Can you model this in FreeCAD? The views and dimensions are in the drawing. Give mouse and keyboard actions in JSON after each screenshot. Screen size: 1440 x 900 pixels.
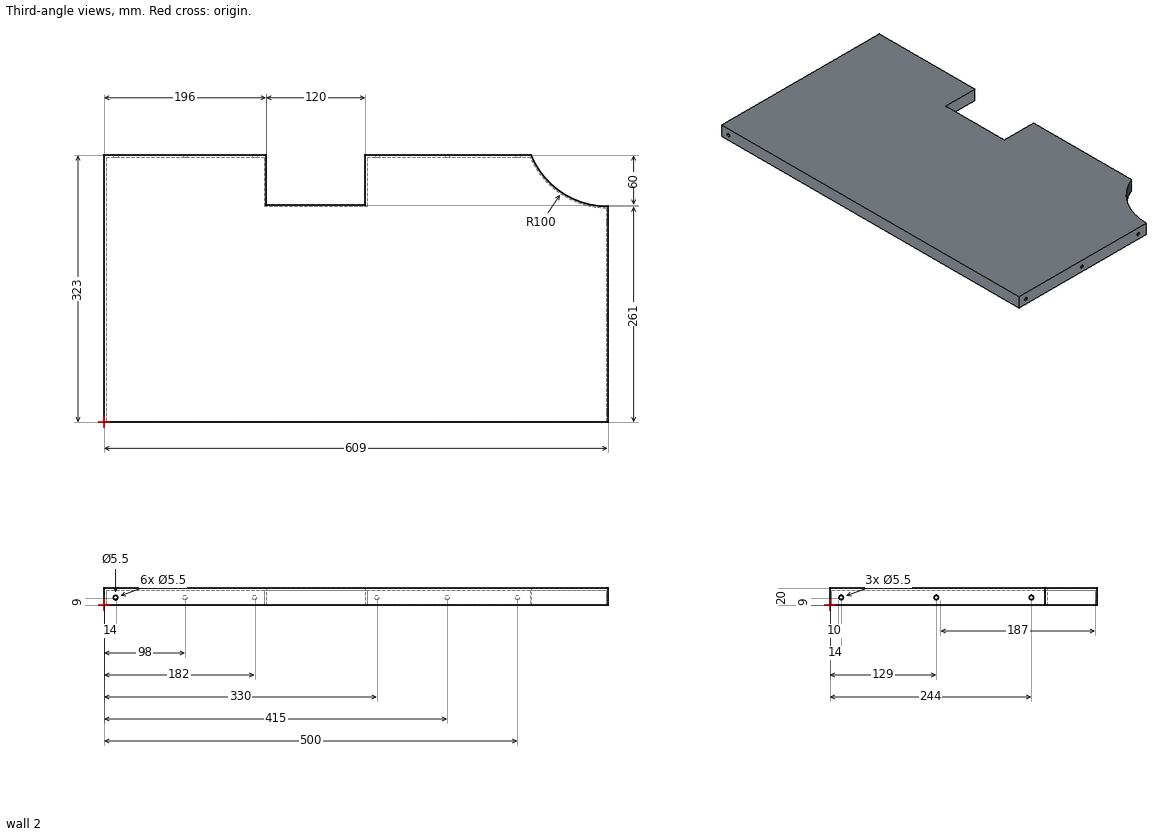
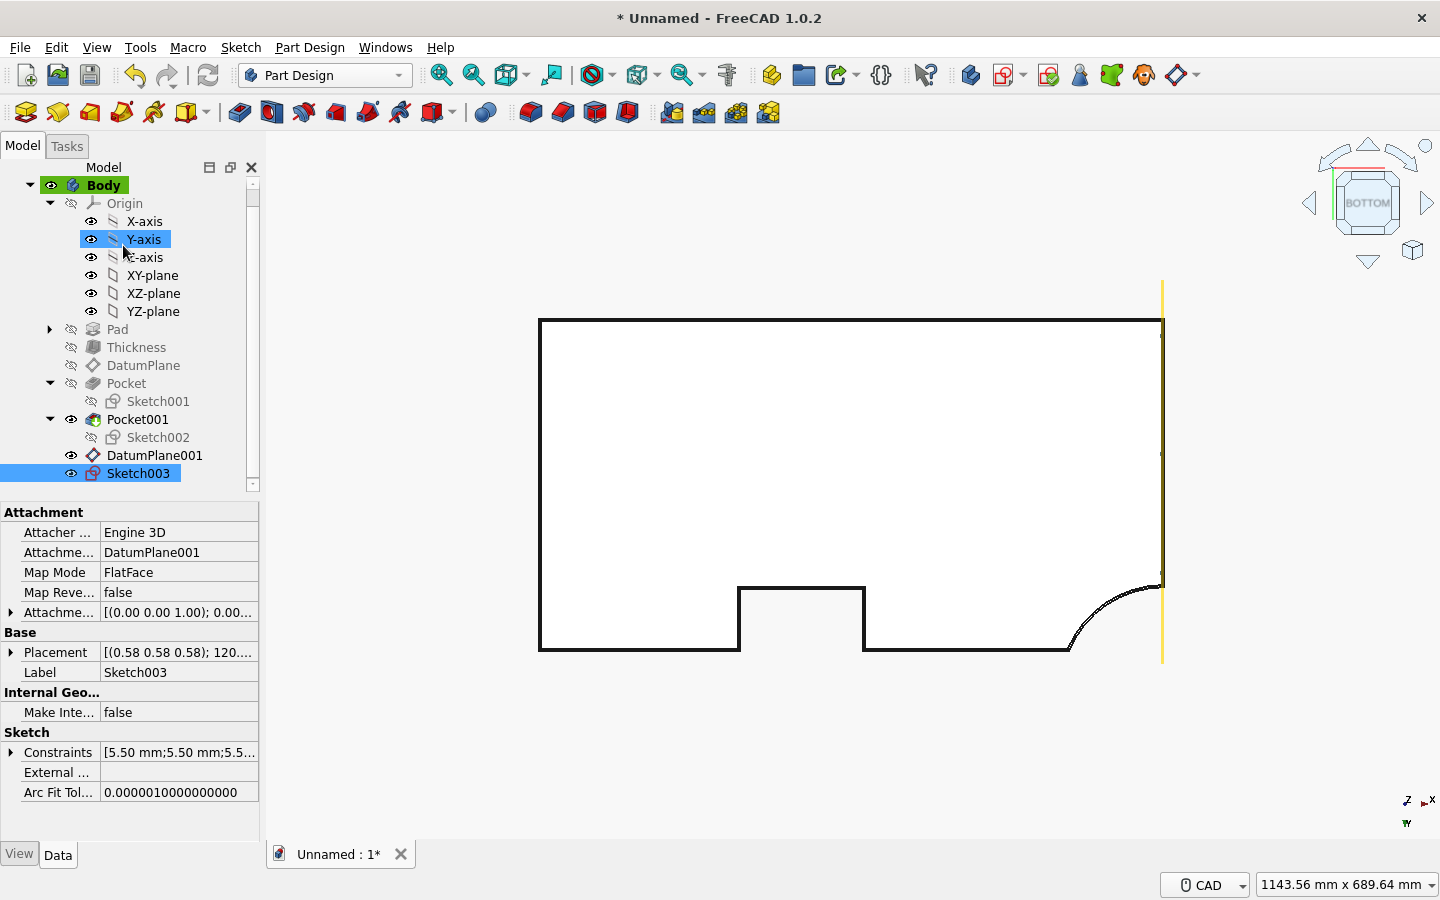
{"action": "left_click", "coordinate": [240, 112]}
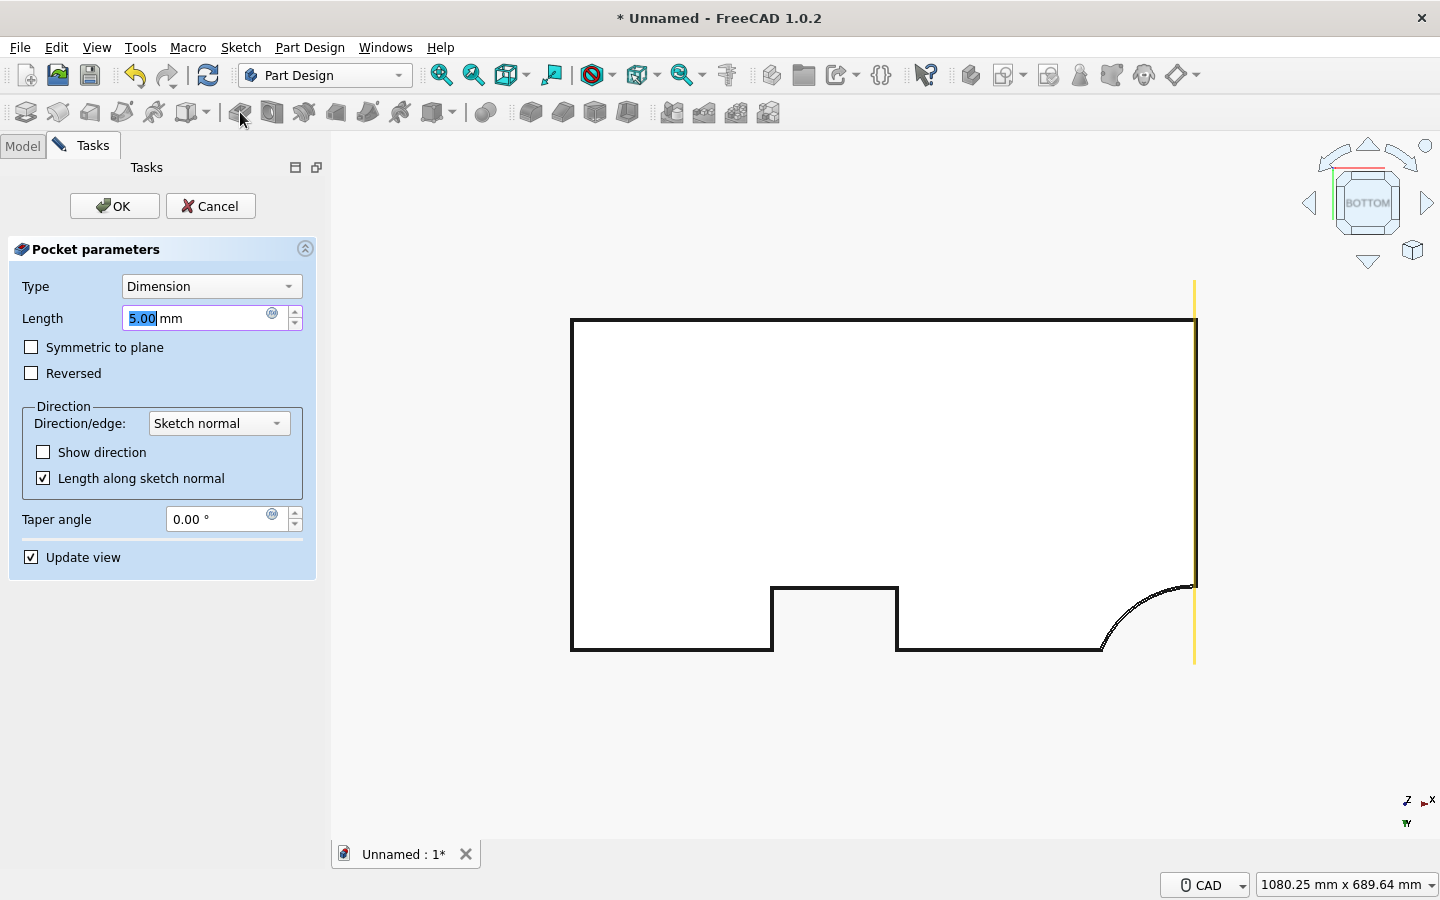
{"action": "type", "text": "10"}
{"action": "key", "text": "Tab"}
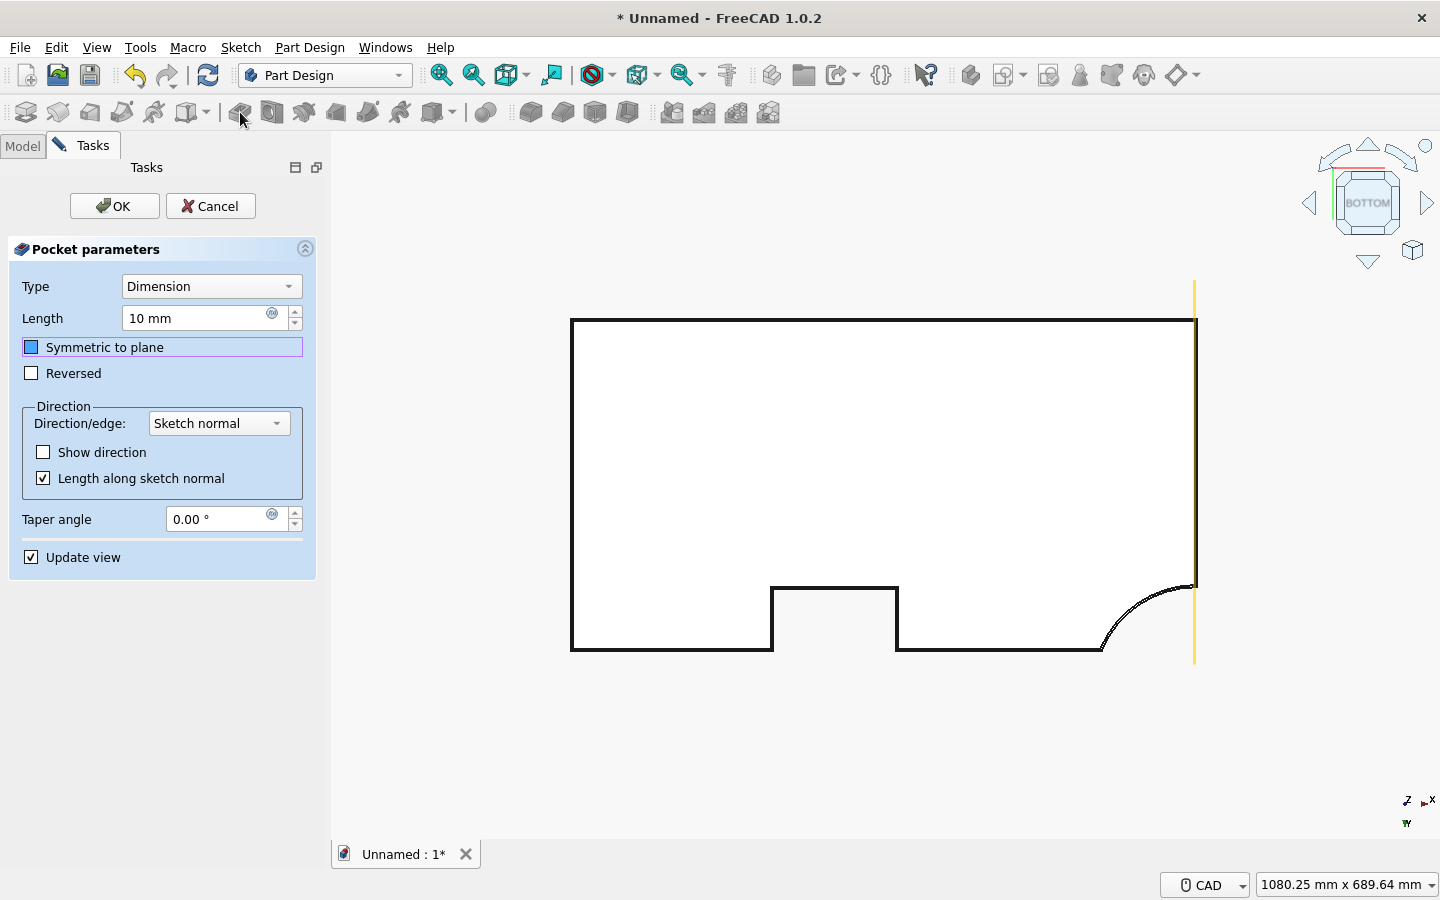
{"action": "left_click", "coordinate": [30, 373]}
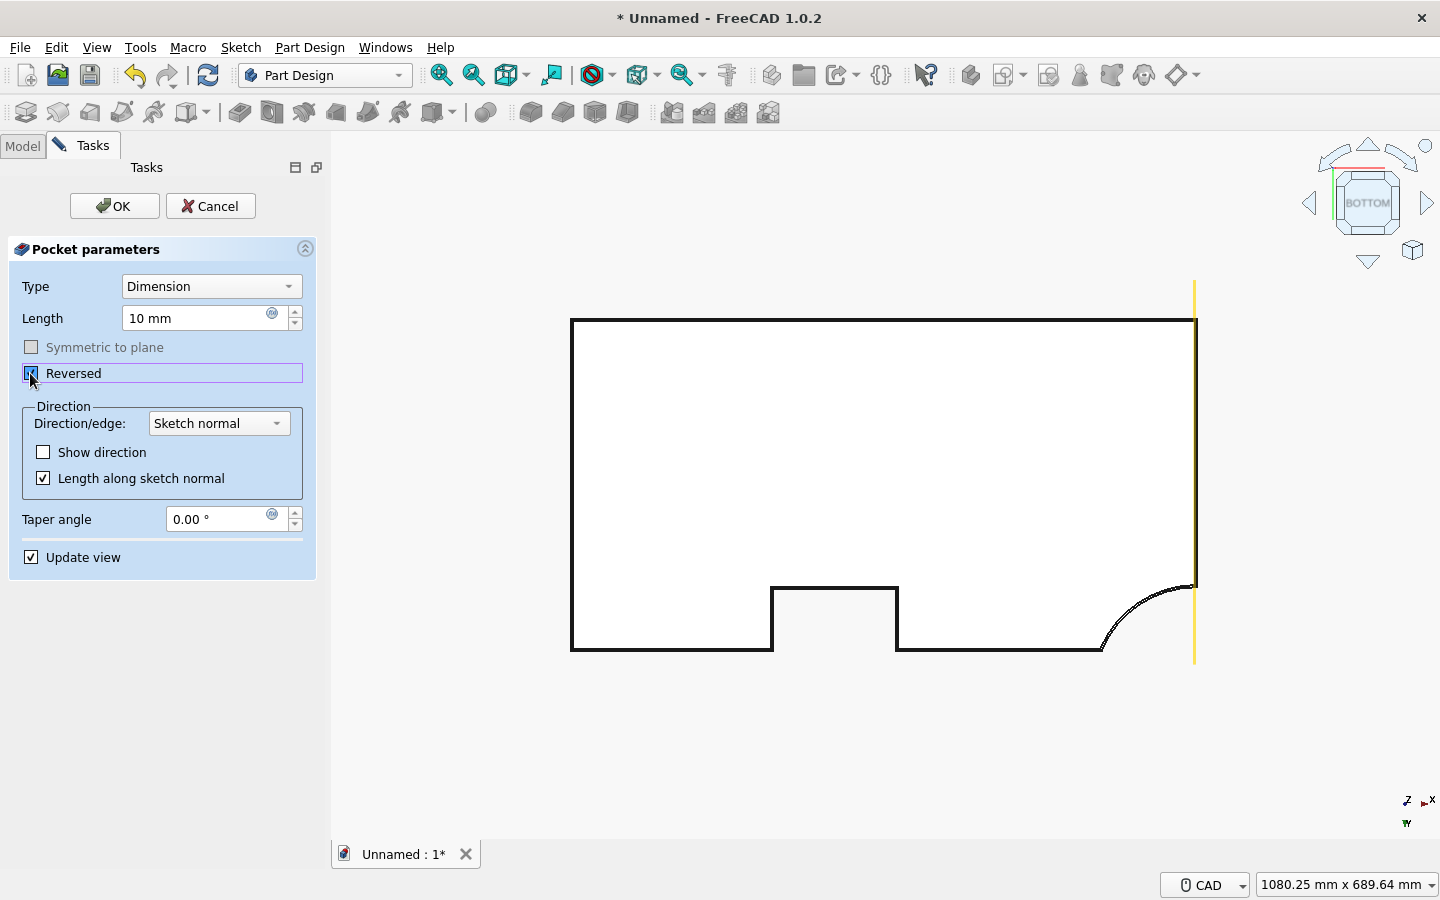
{"action": "left_click", "coordinate": [115, 206]}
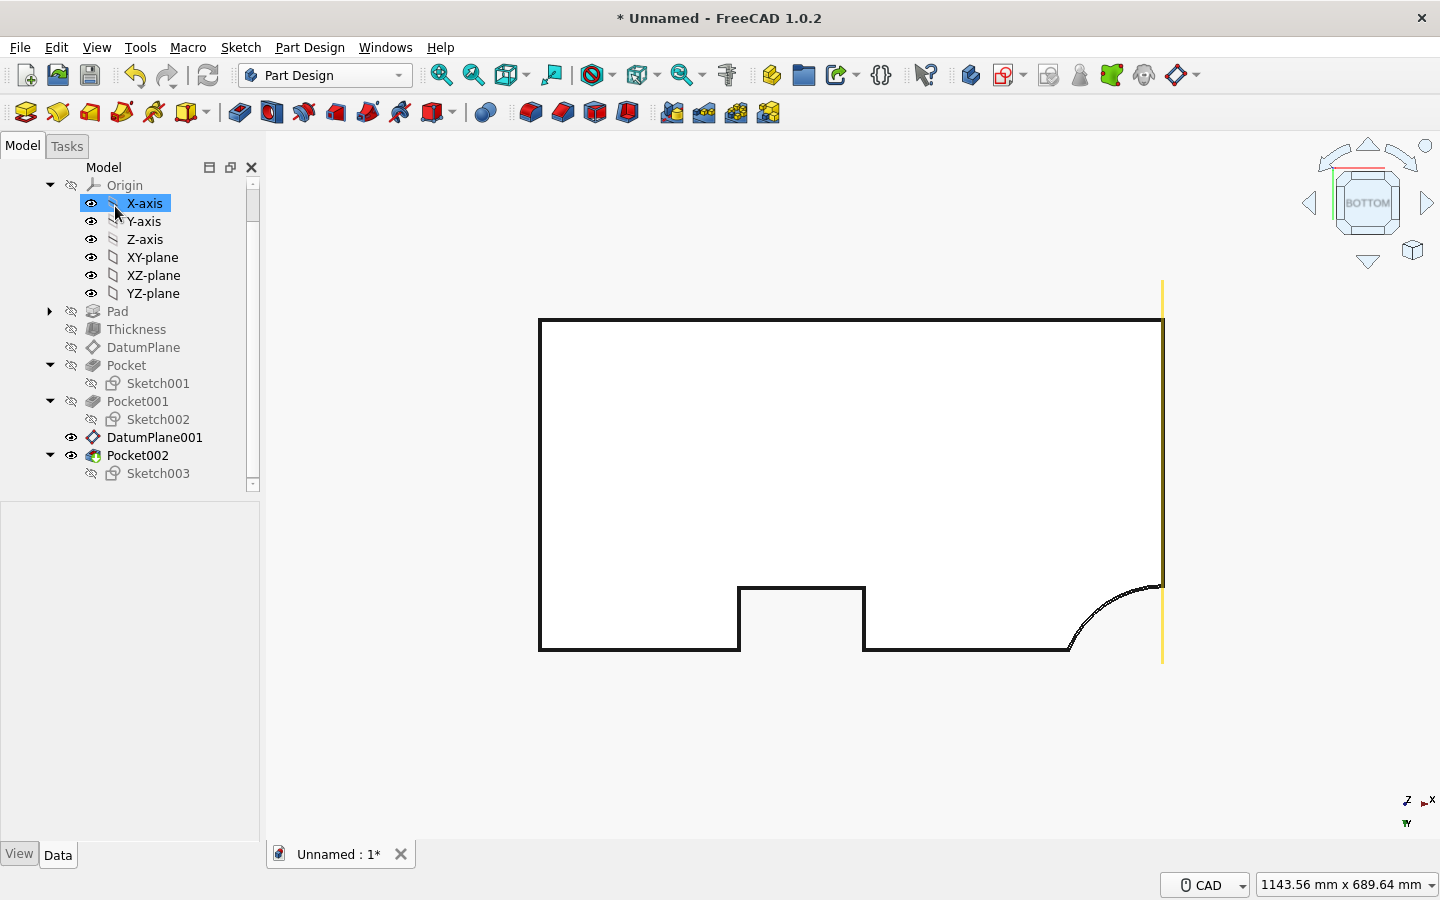
{"action": "left_click", "coordinate": [116, 437]}
{"action": "key", "text": "space"}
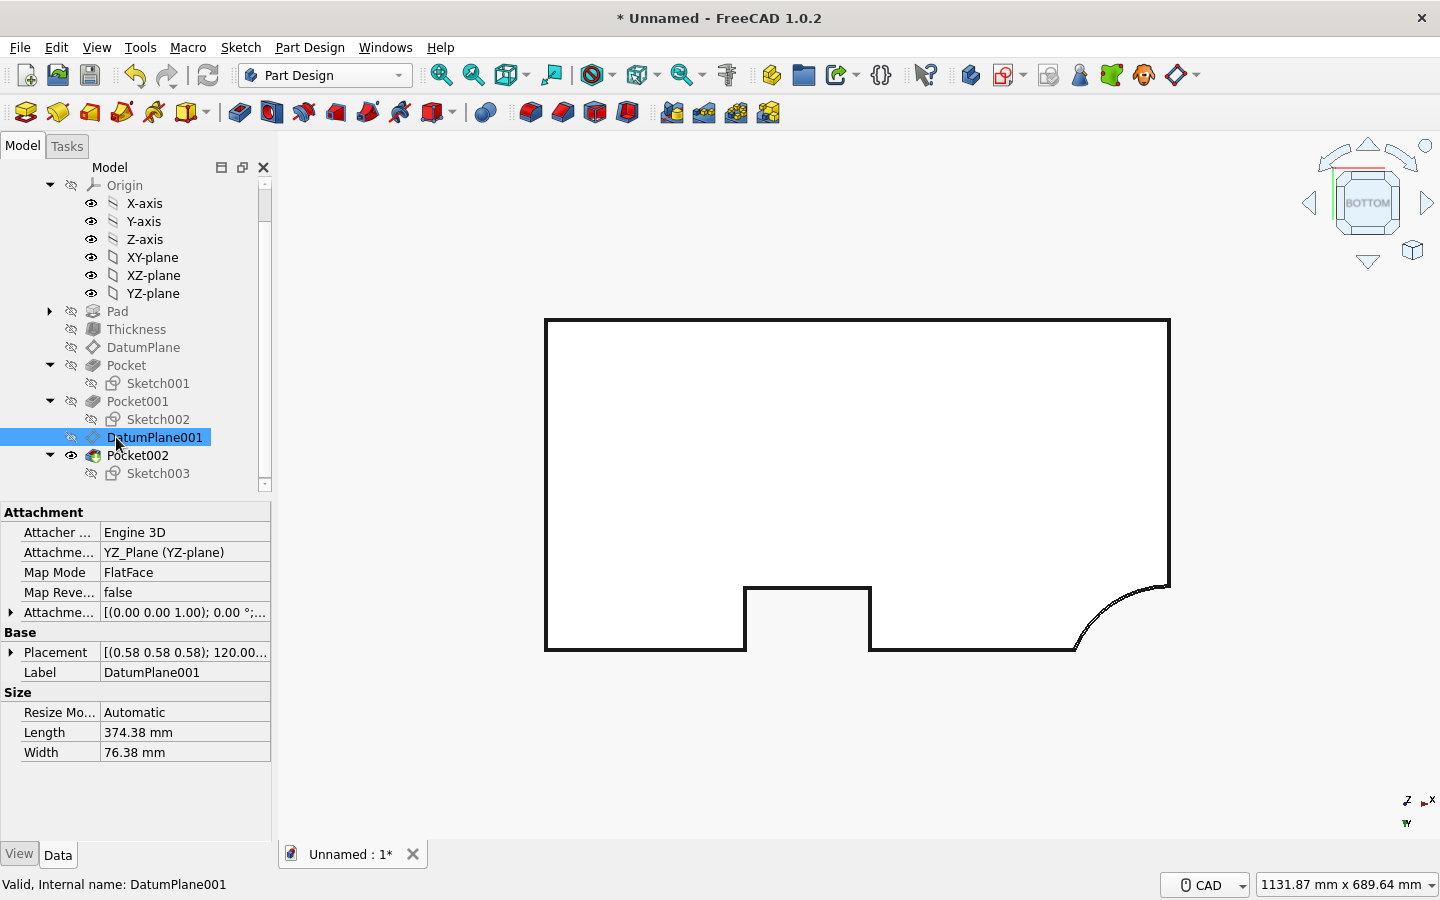
{"action": "key", "text": "0"}